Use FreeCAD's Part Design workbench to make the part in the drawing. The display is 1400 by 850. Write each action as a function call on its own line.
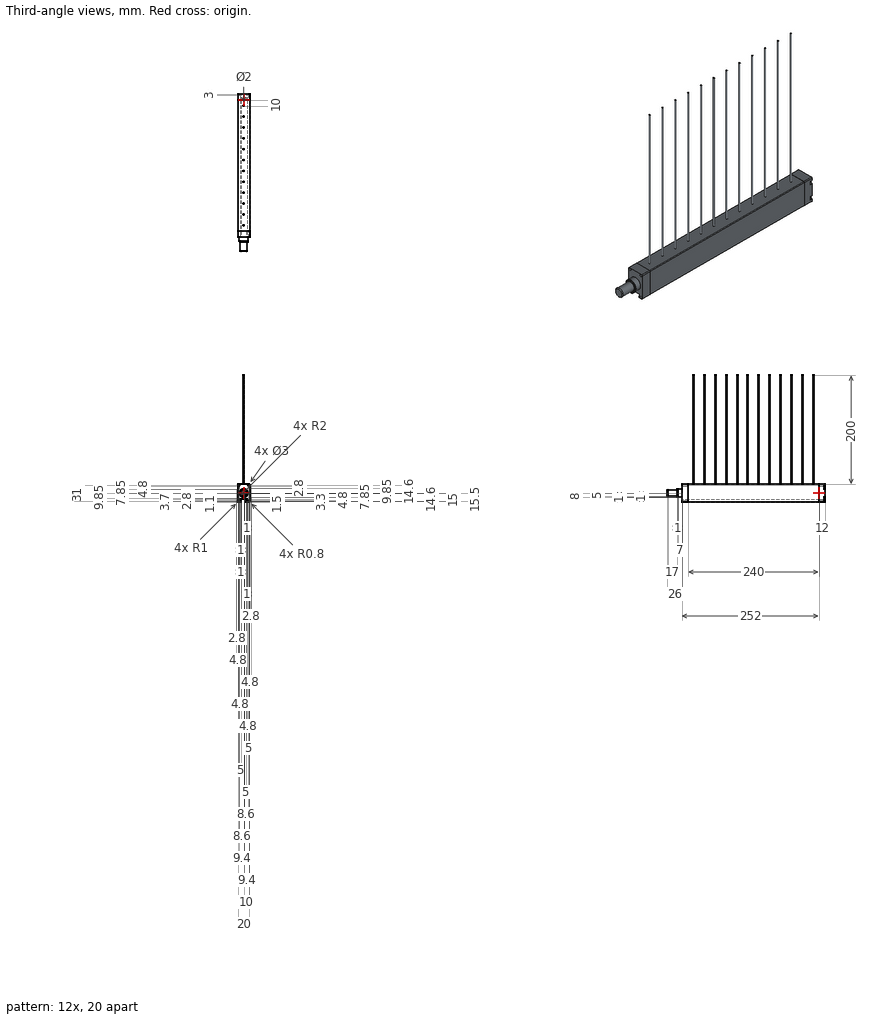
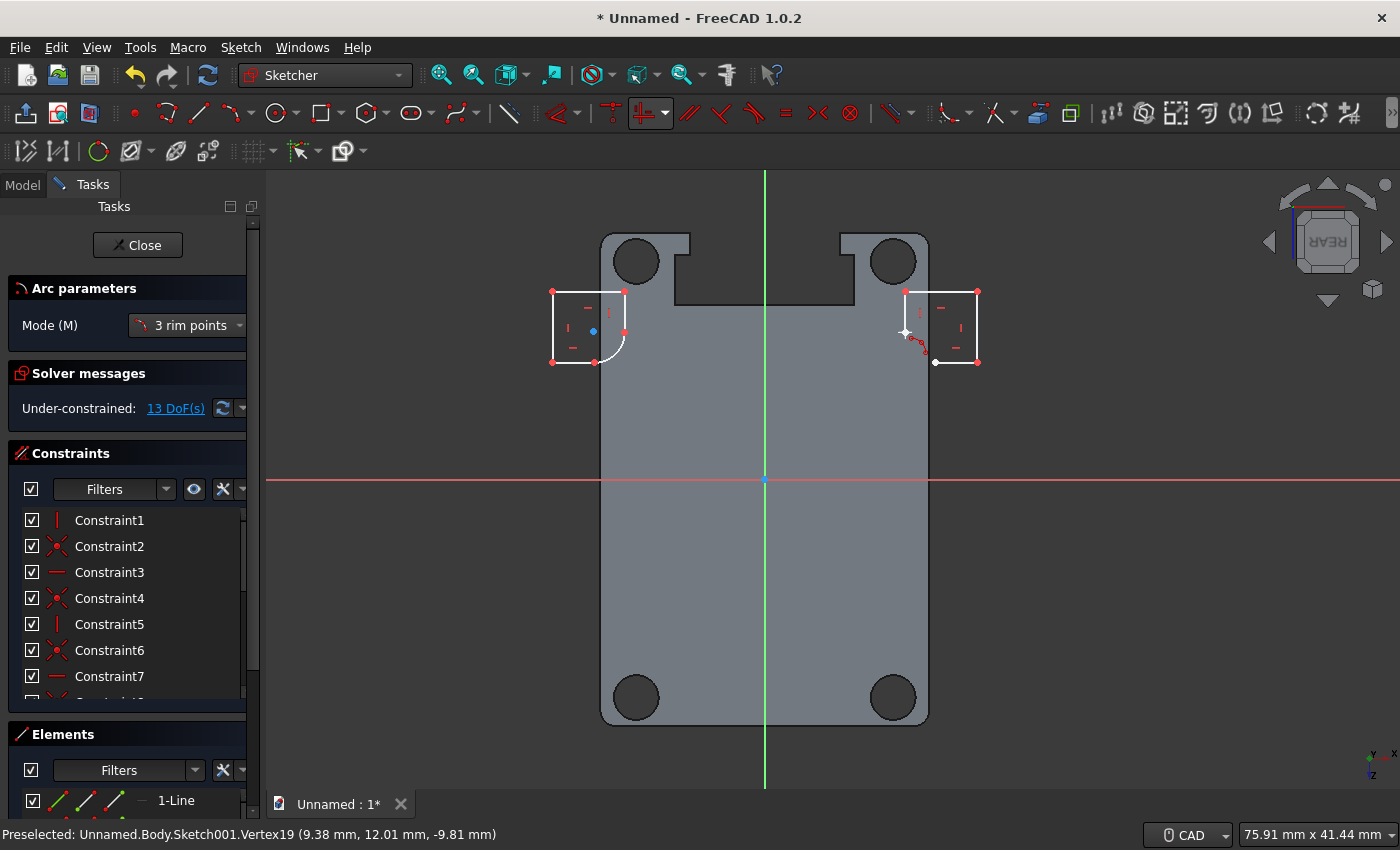
click(905, 333)
click(935, 363)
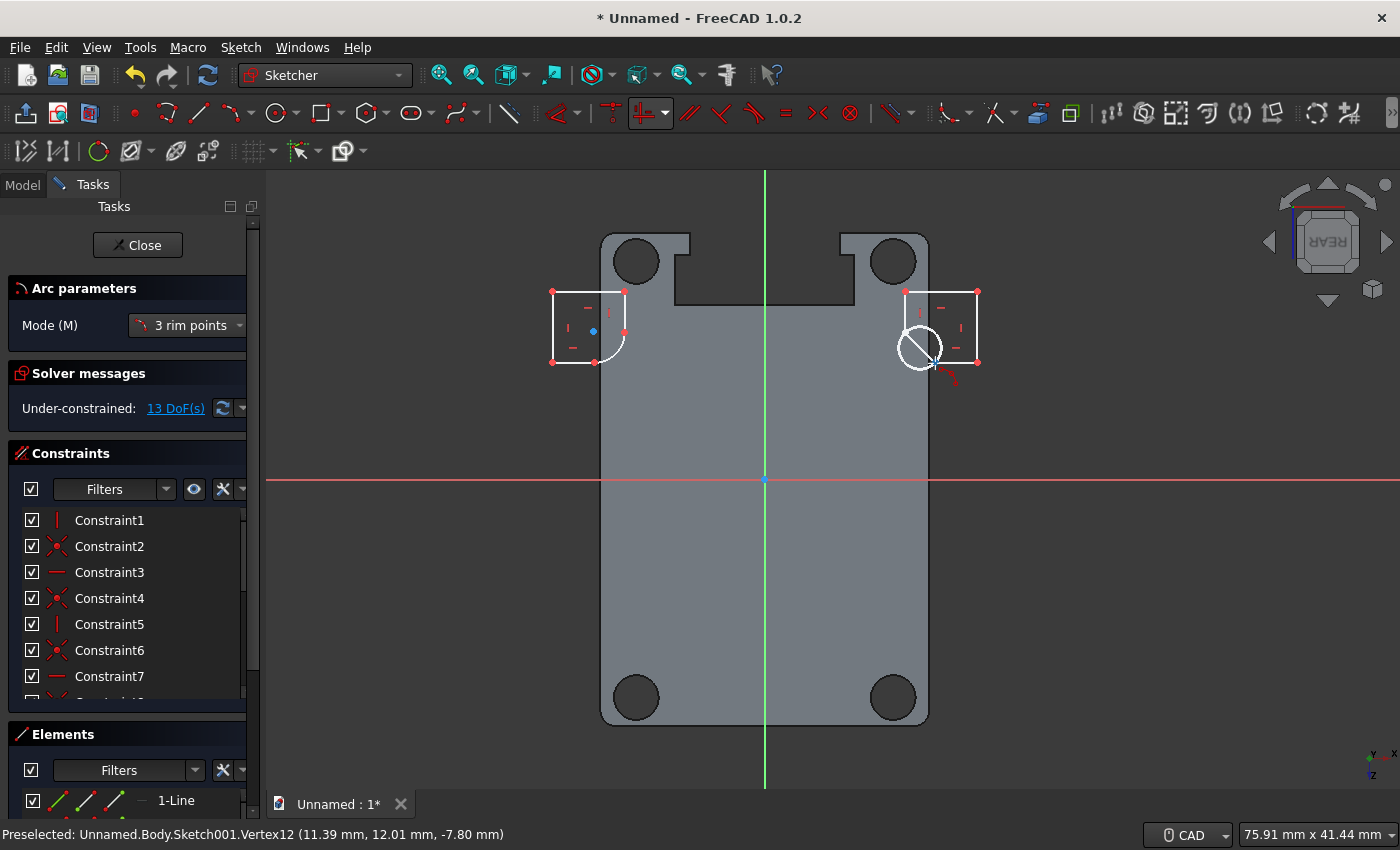
scroll(914, 353, up, 3)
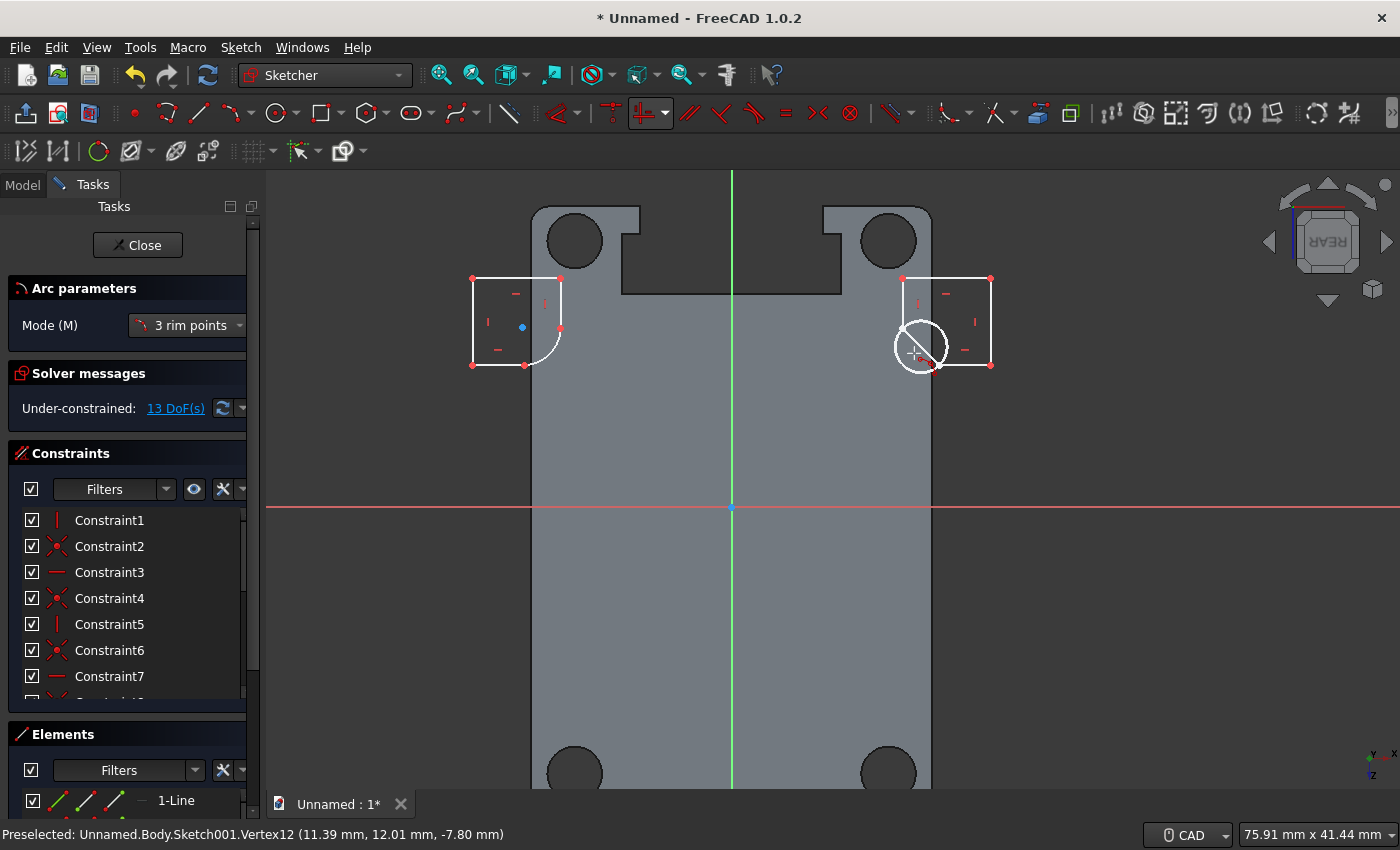
click(913, 354)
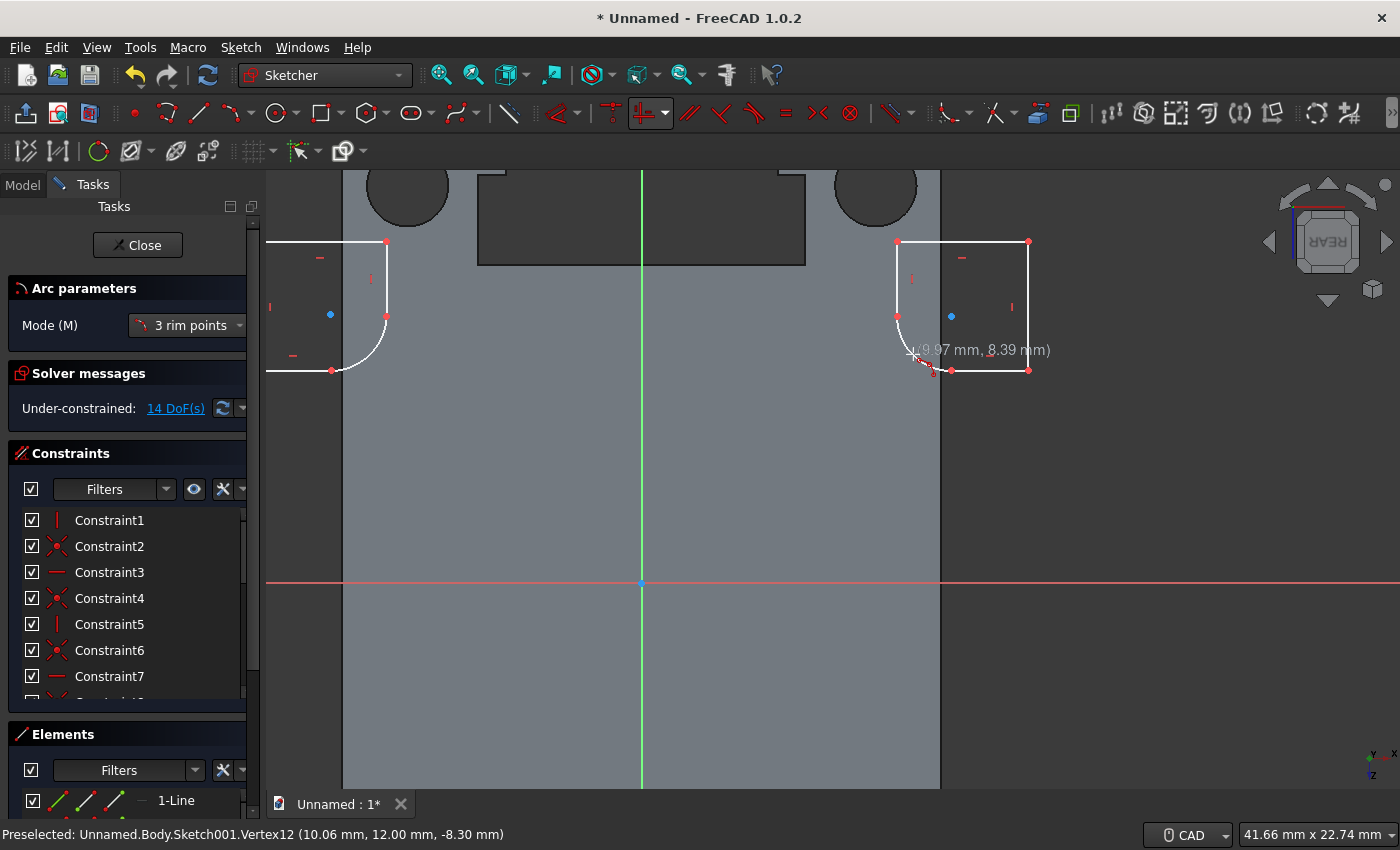
click(168, 114)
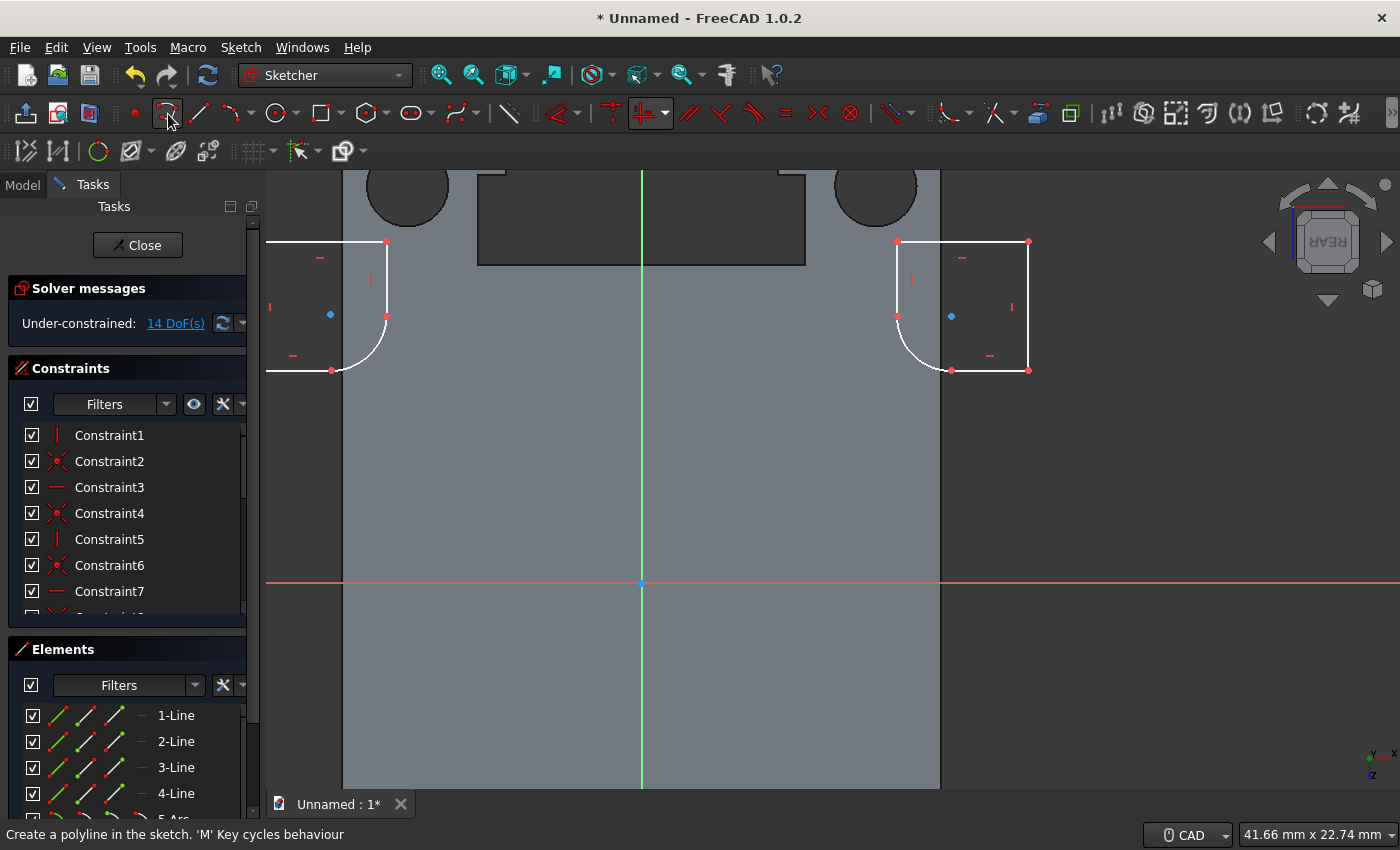
scroll(914, 353, down, 3)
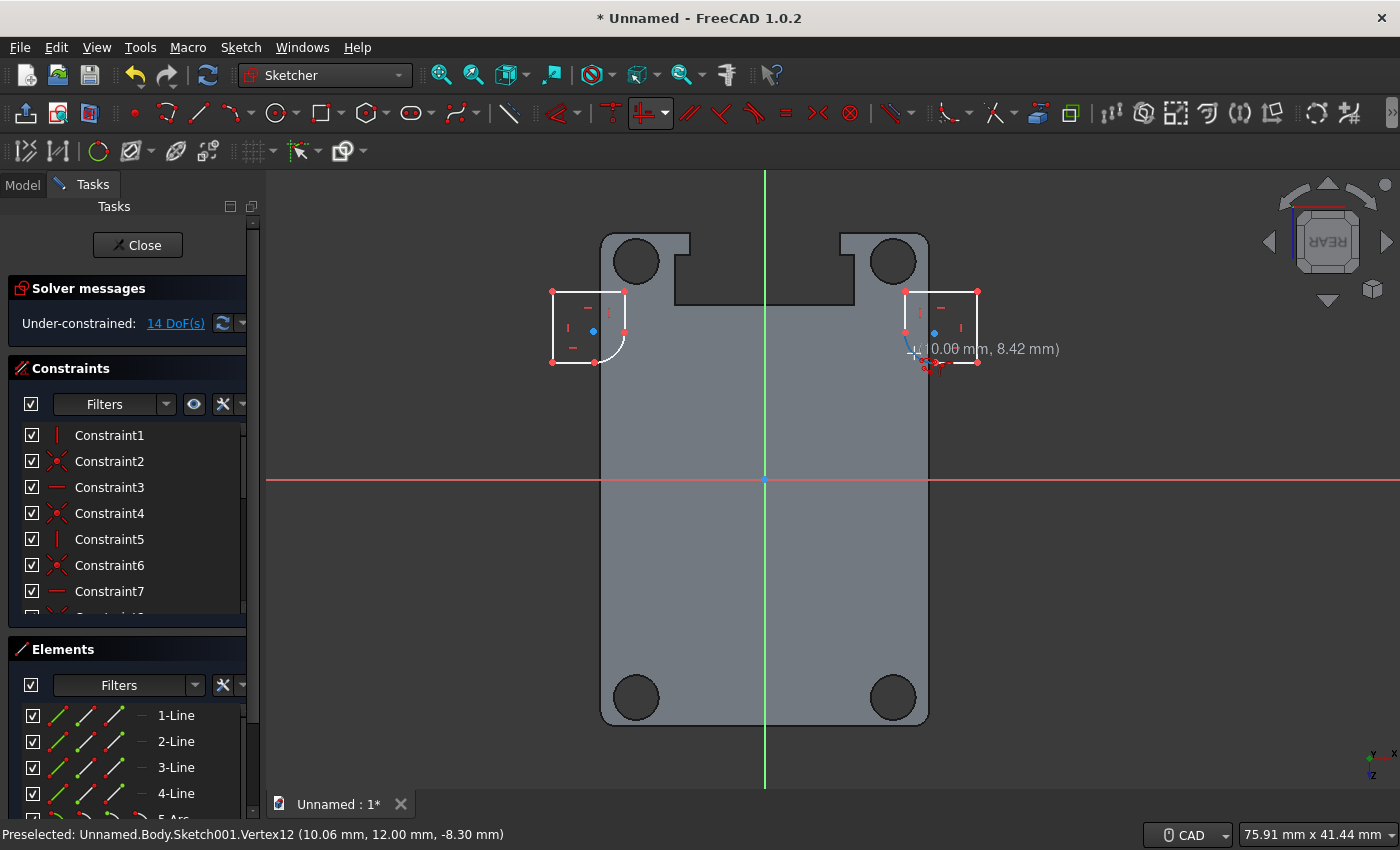
click(905, 627)
click(905, 668)
click(977, 668)
click(977, 597)
click(935, 597)
right_click(935, 597)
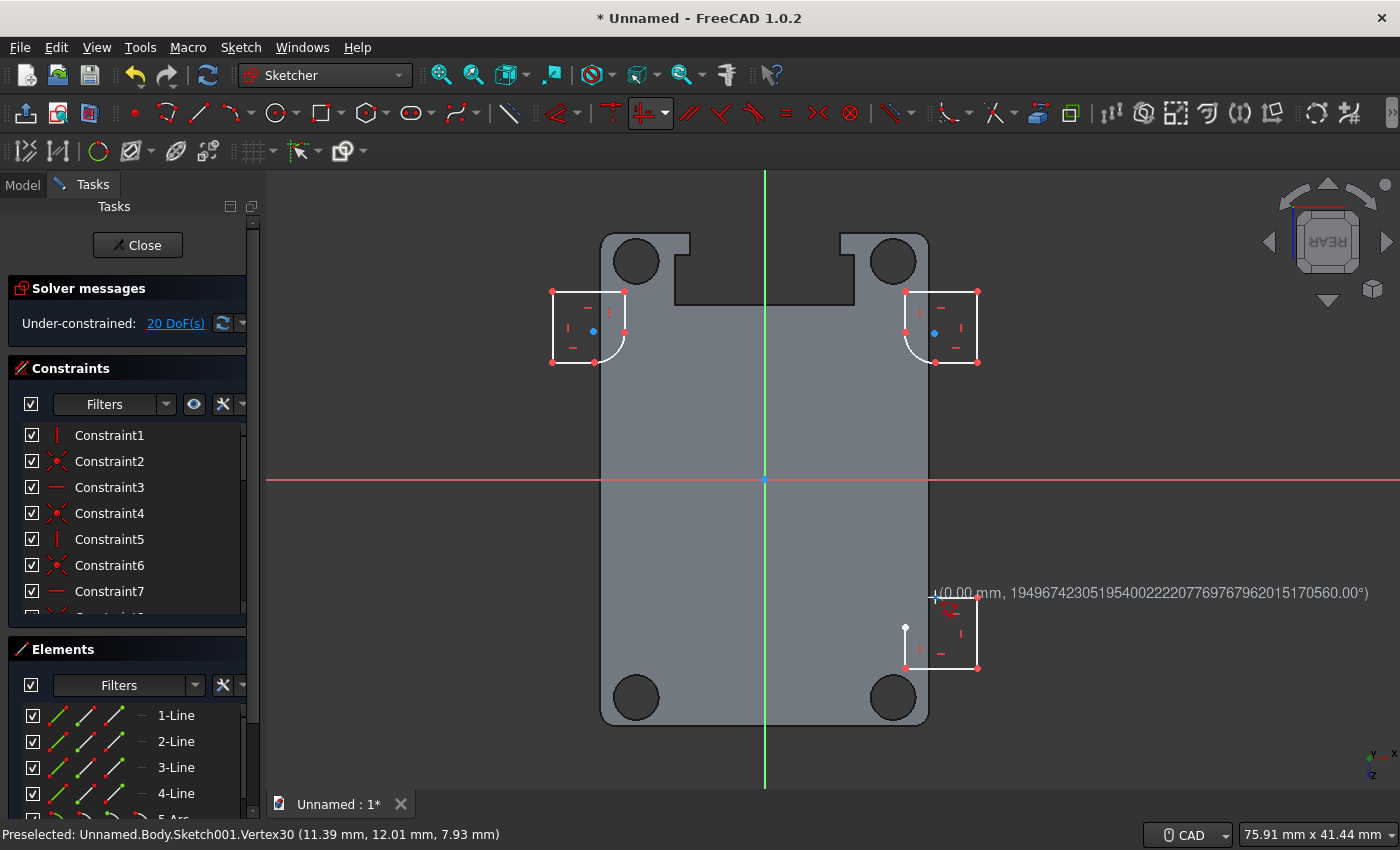
click(232, 114)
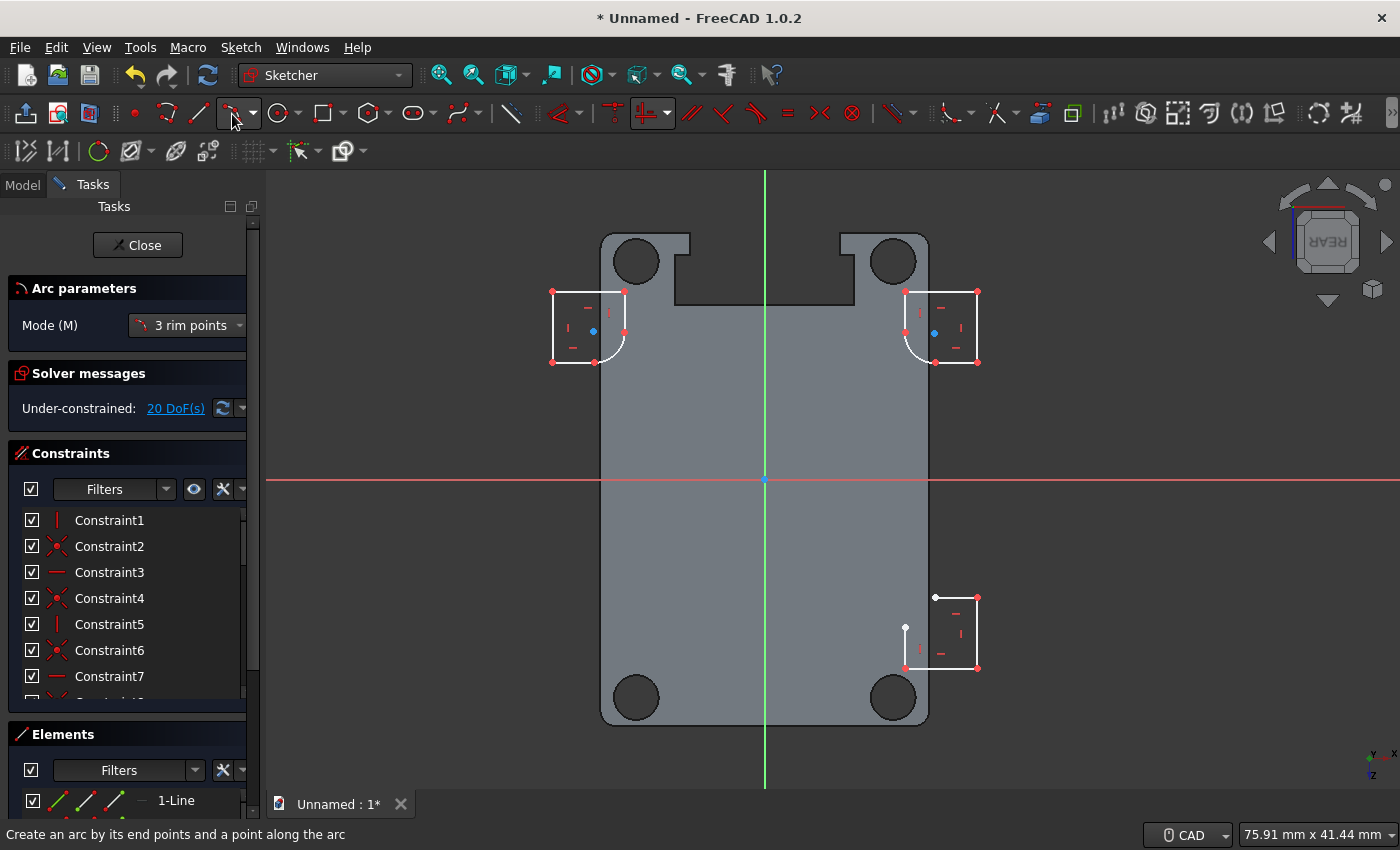
click(935, 598)
click(905, 628)